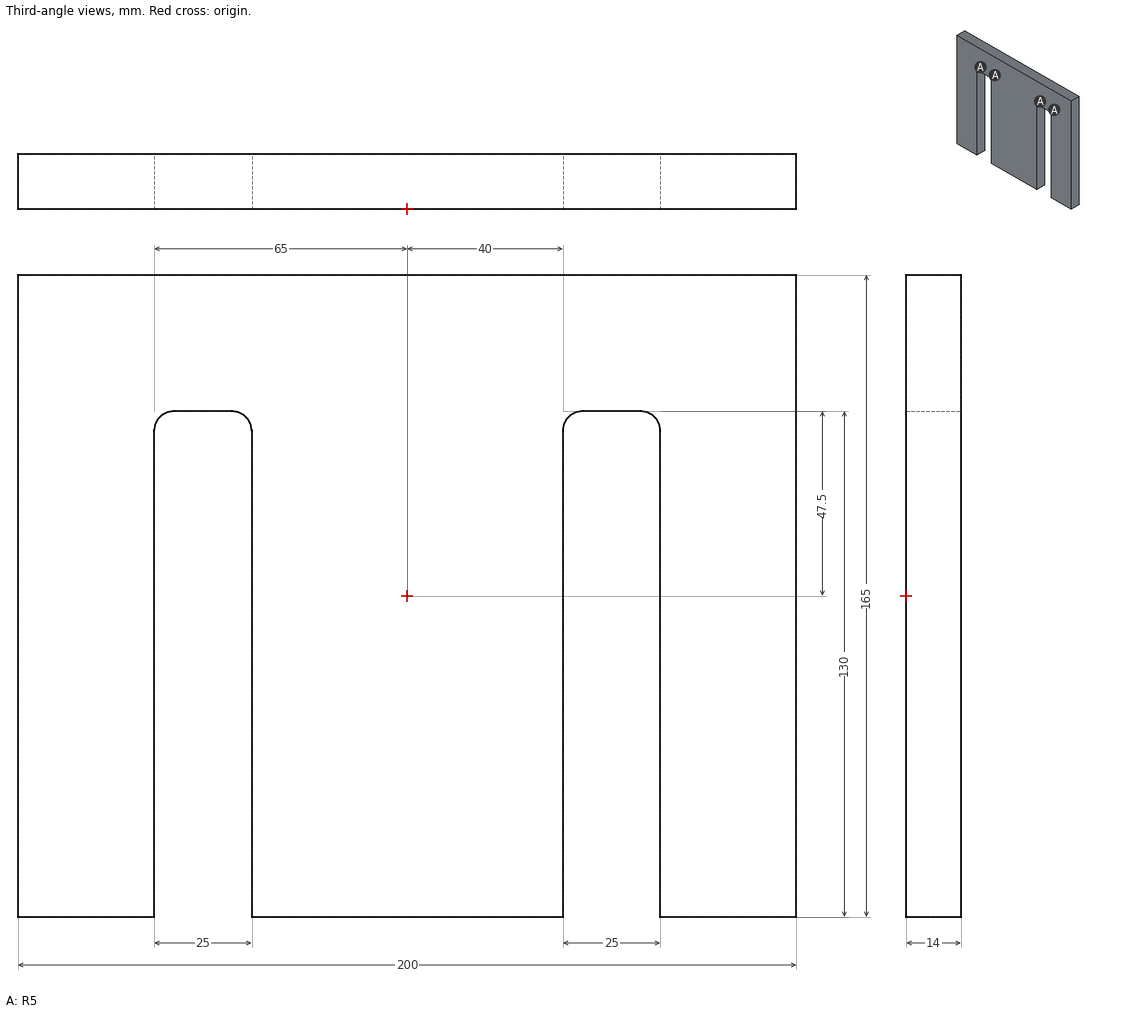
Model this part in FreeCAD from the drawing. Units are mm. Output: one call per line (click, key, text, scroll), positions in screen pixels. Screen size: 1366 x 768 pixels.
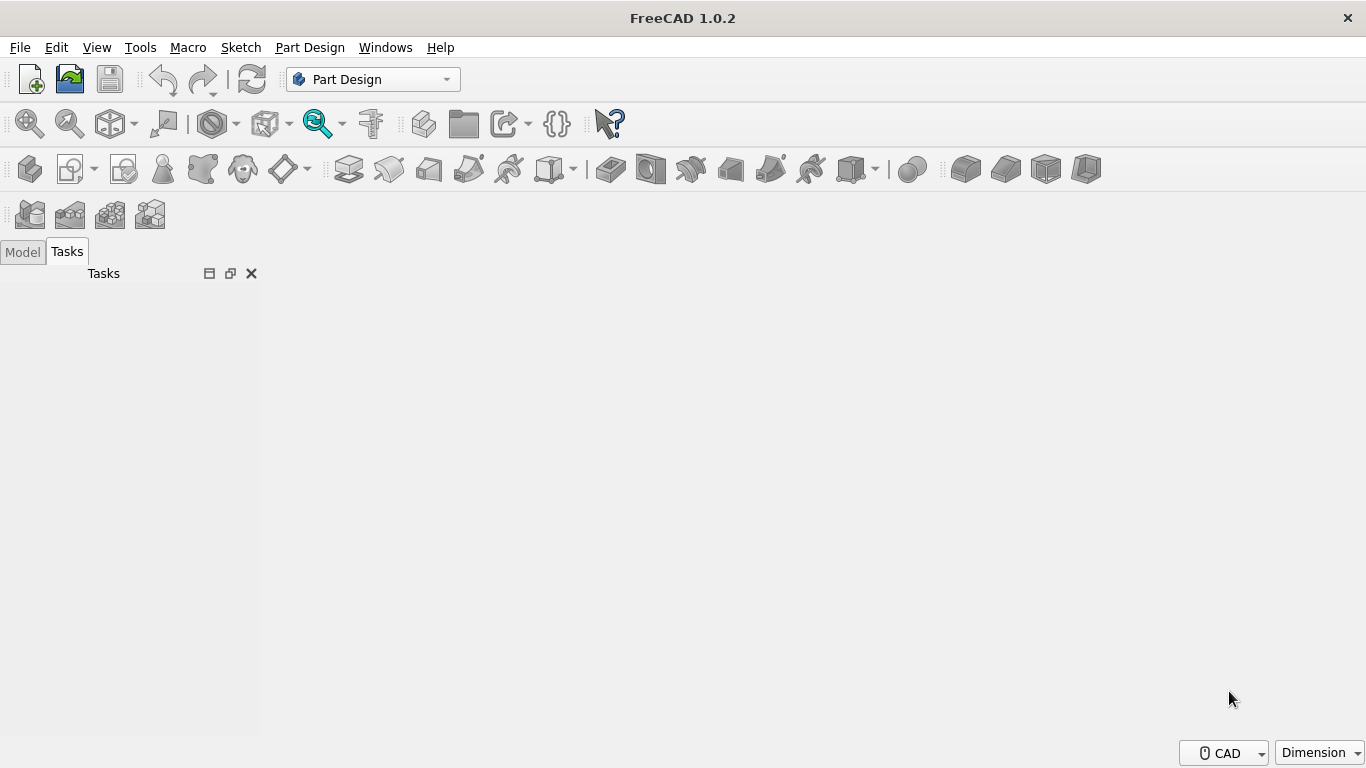
click(30, 80)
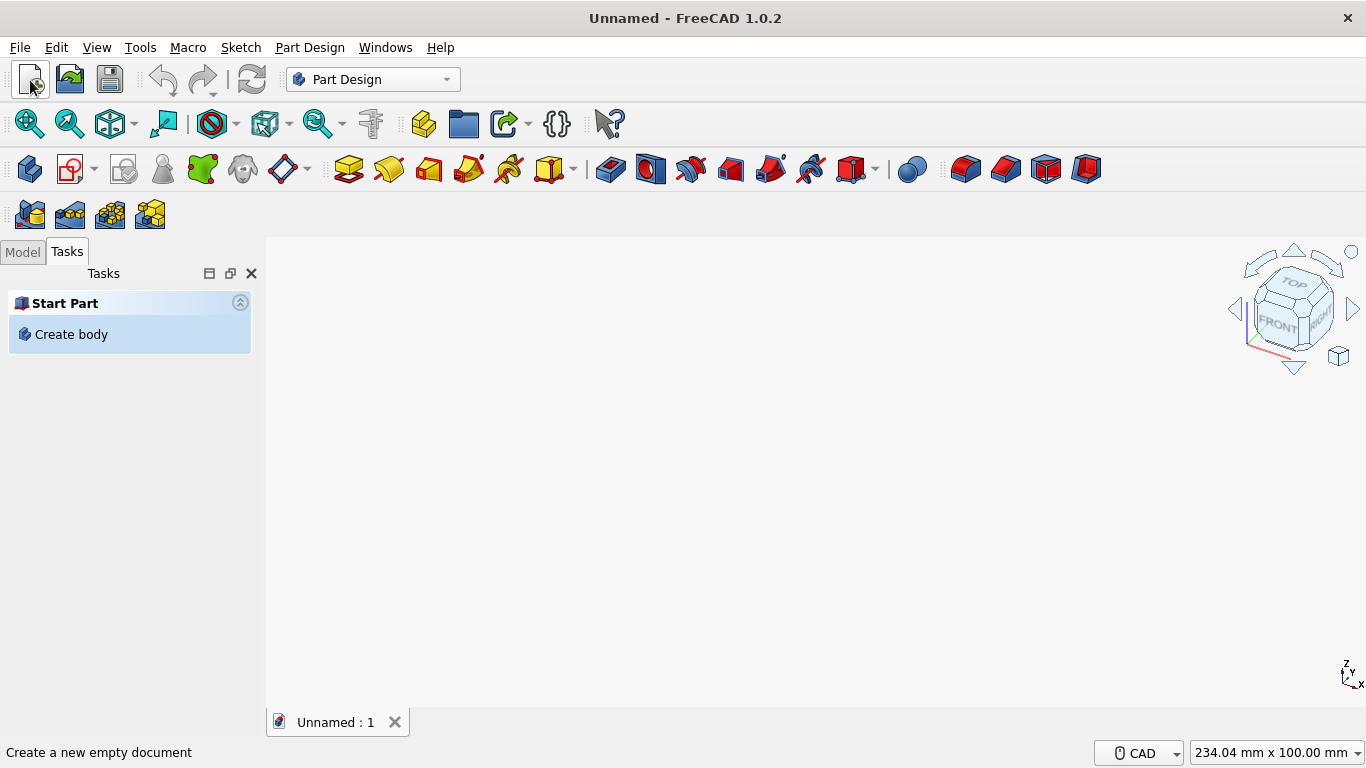
click(70, 170)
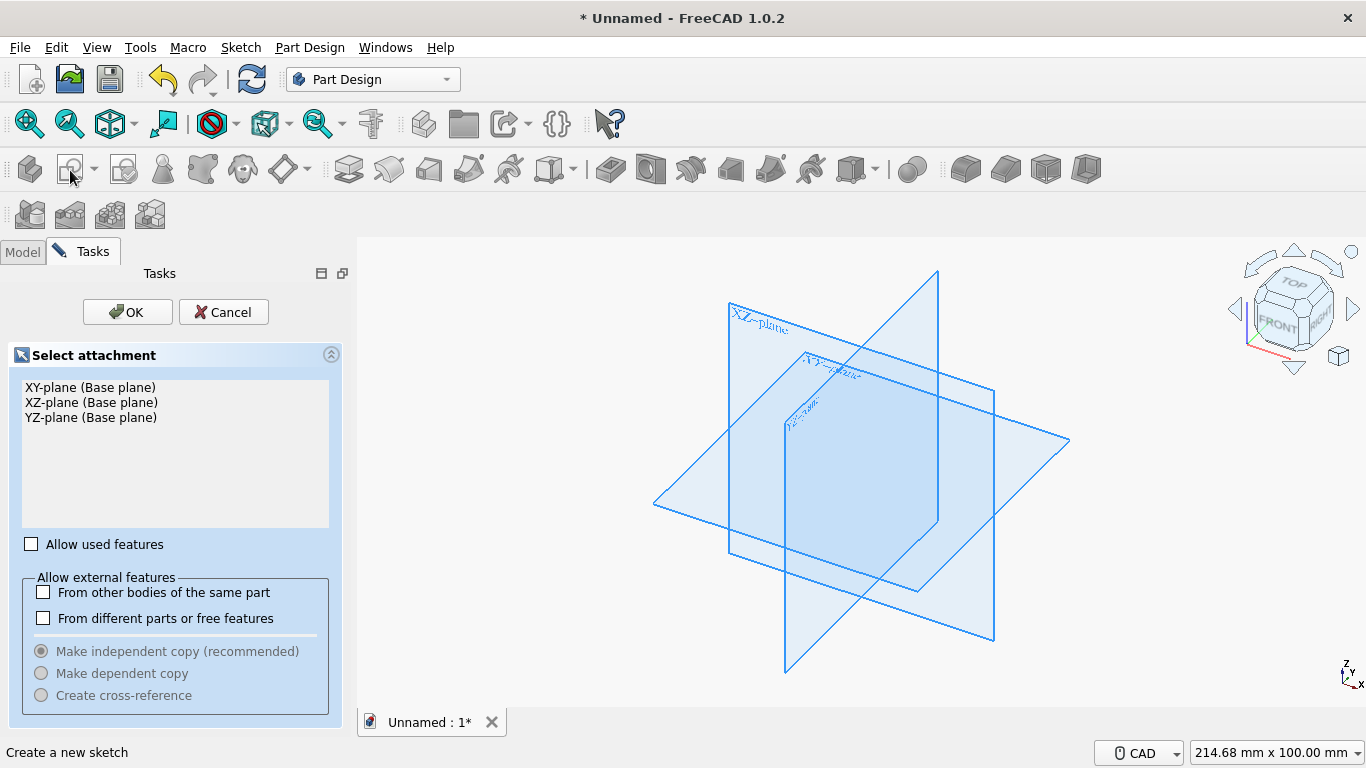
click(82, 402)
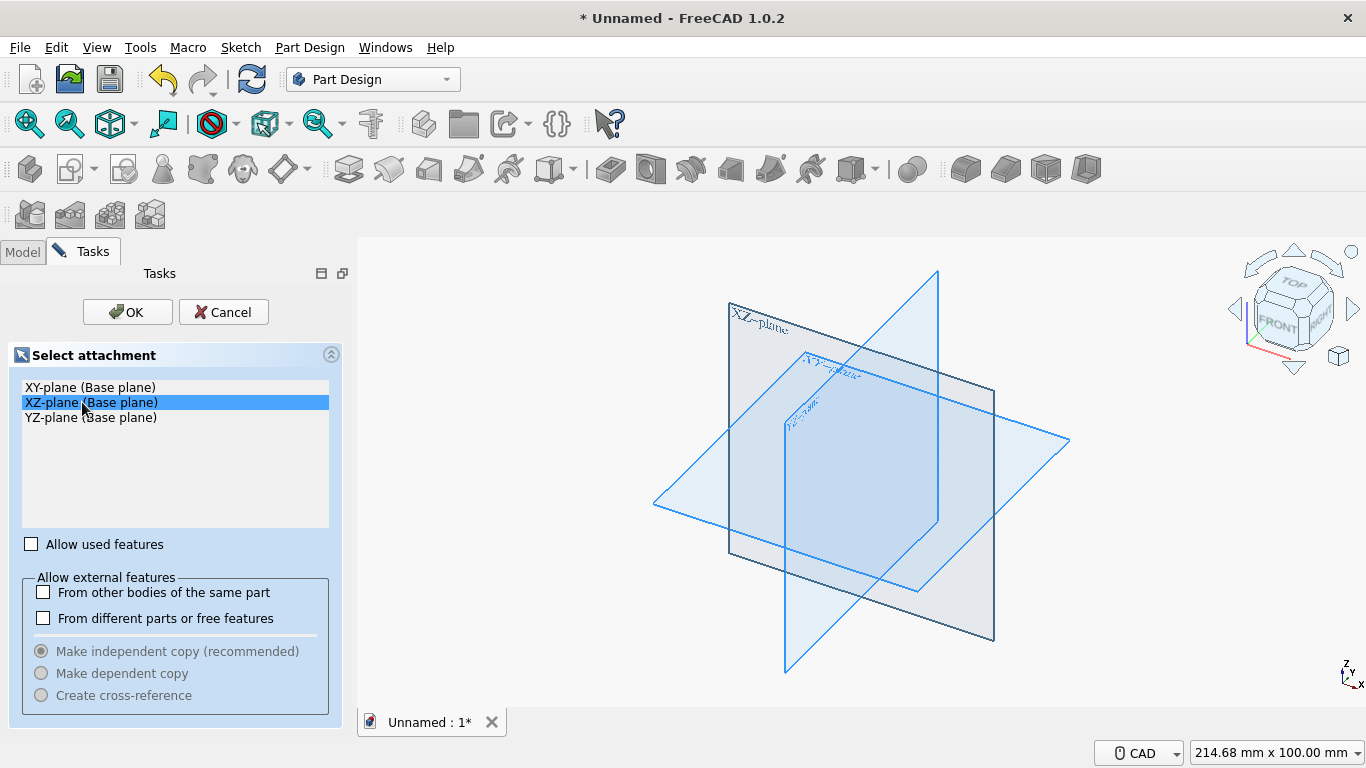
click(128, 312)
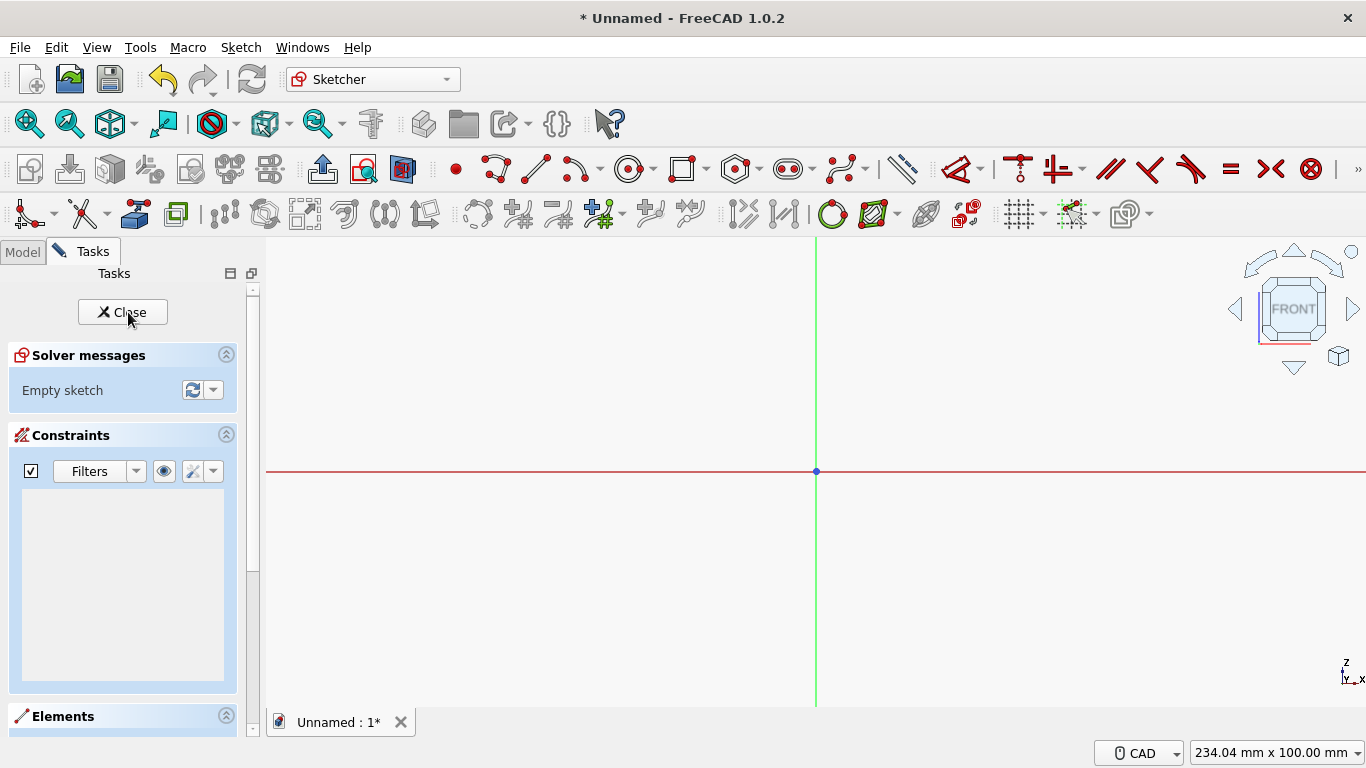
scroll(708, 472, down, 5)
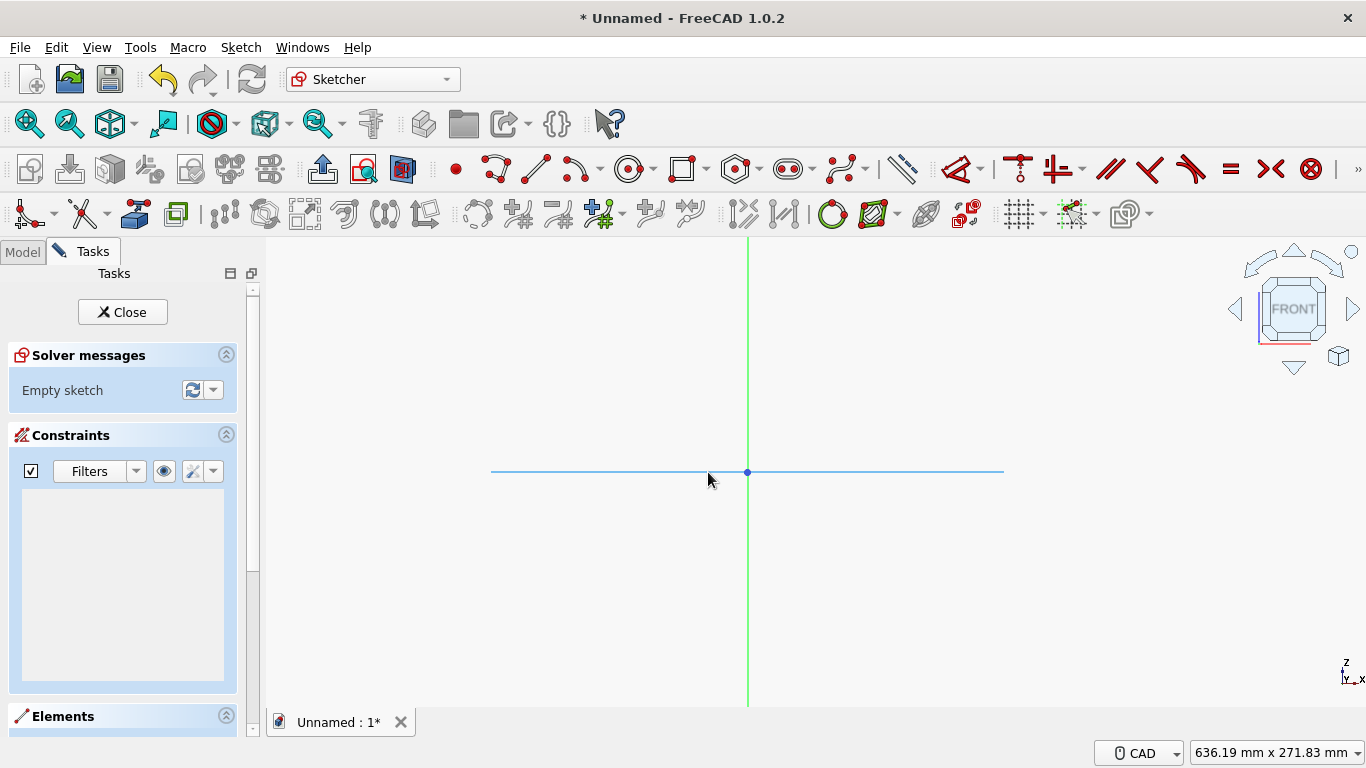
key(g)
key(v)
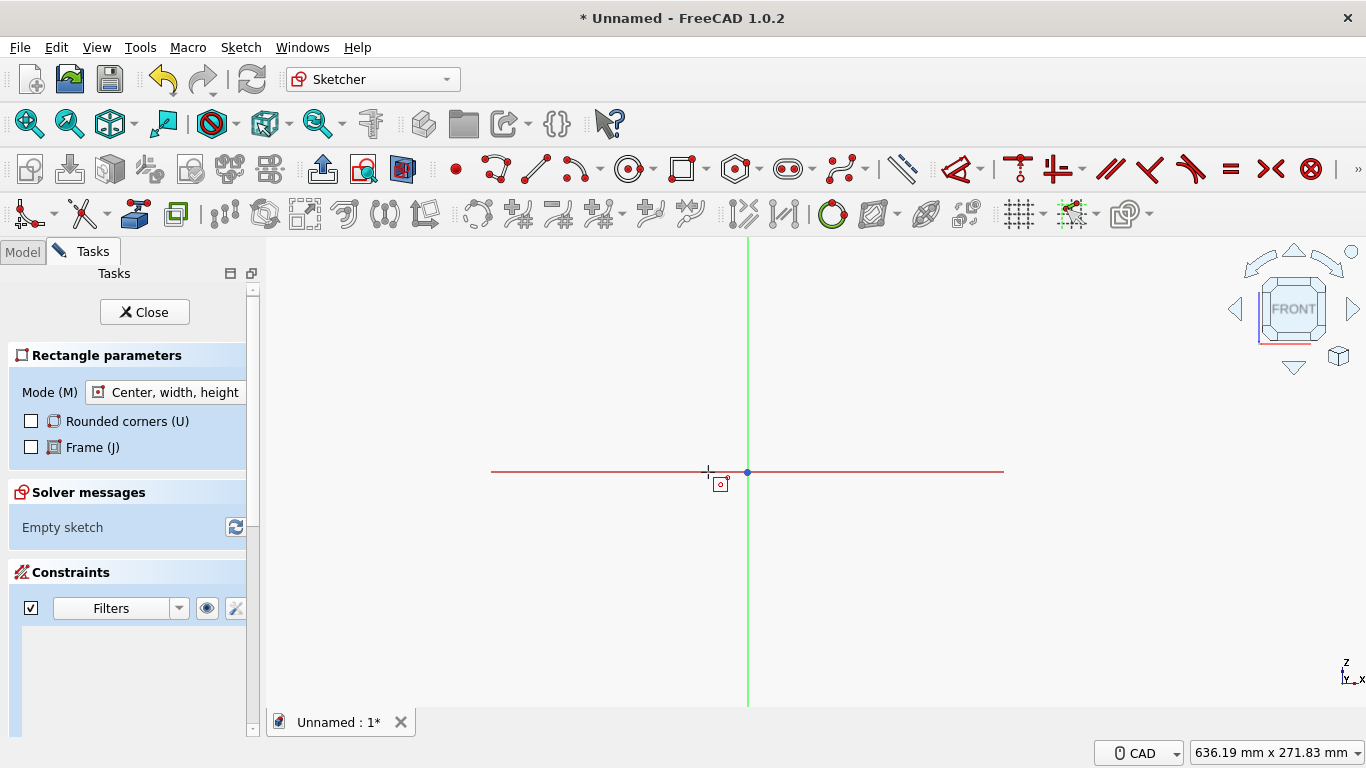
click(748, 472)
move(921, 330)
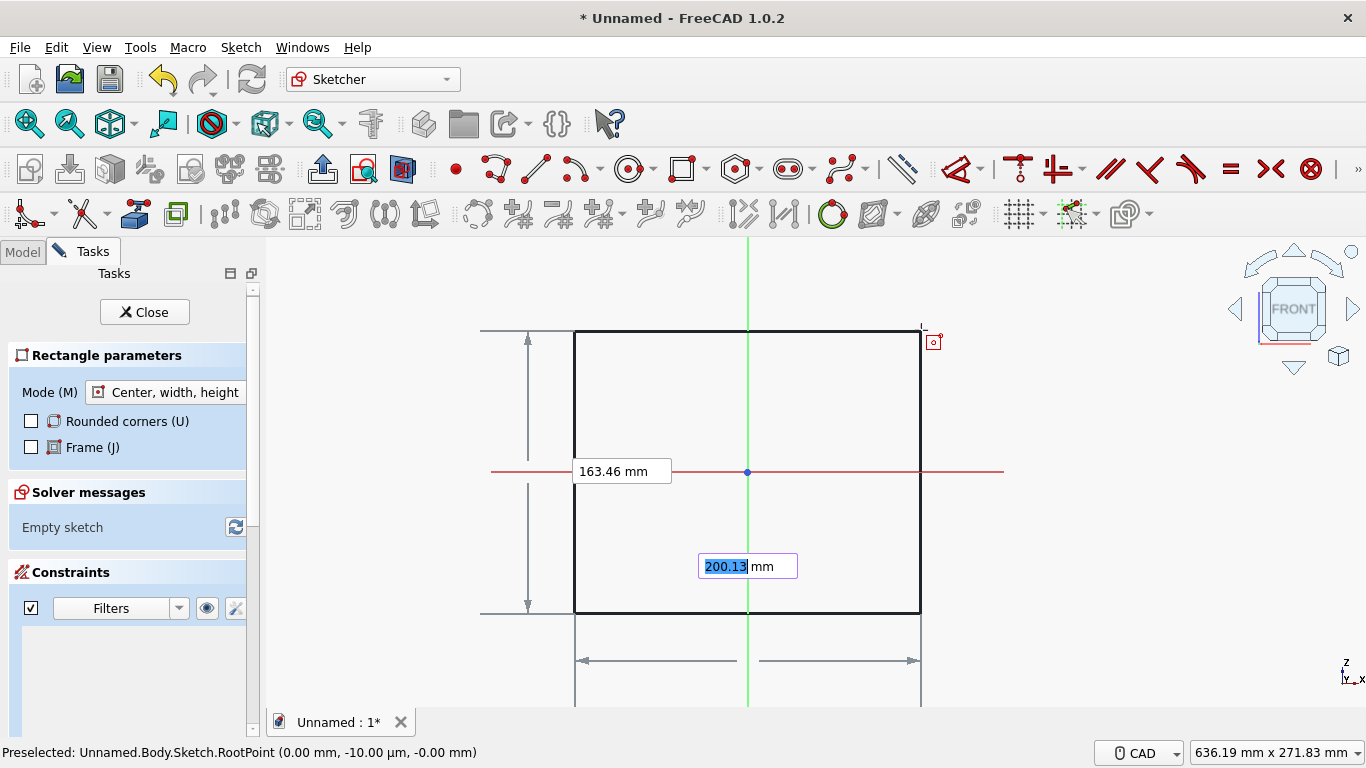
text(200)
key(Tab)
text(165)
key(Return)
key(Escape)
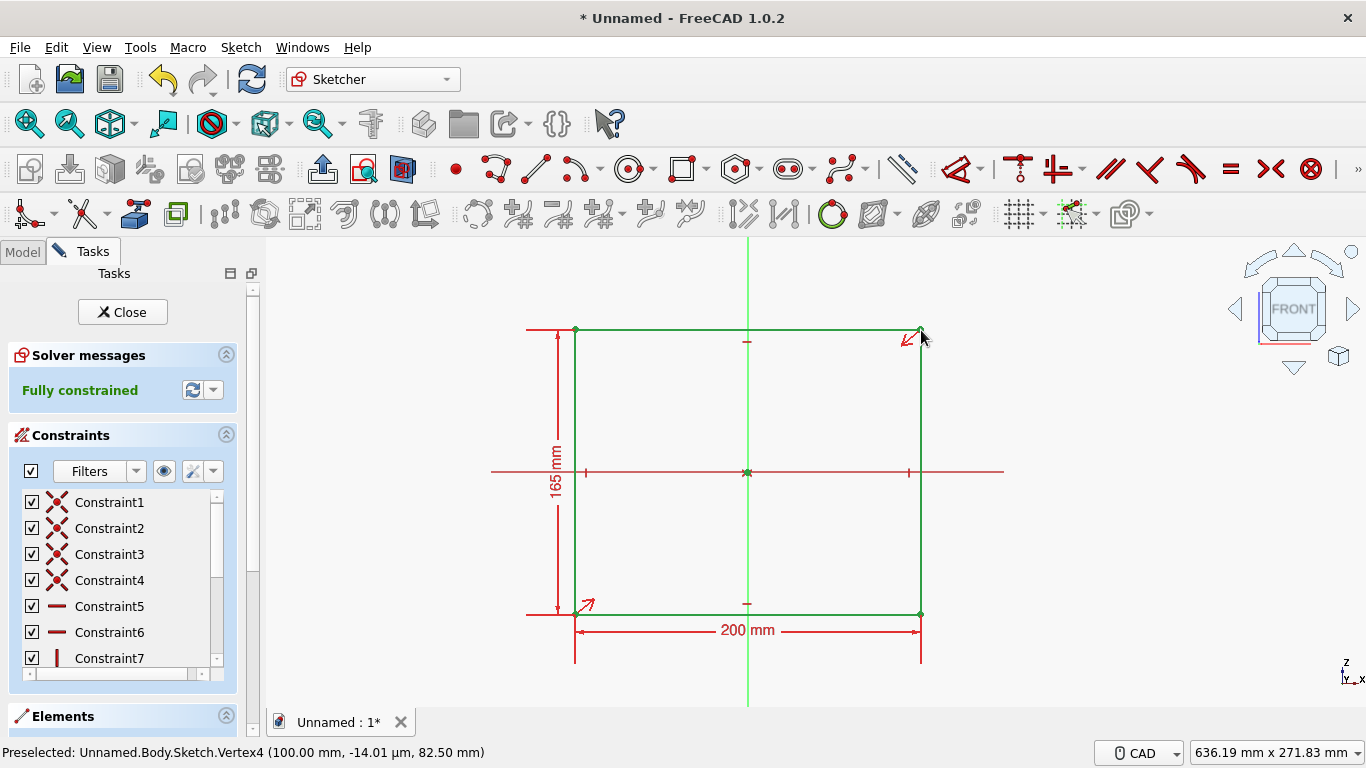
click(123, 312)